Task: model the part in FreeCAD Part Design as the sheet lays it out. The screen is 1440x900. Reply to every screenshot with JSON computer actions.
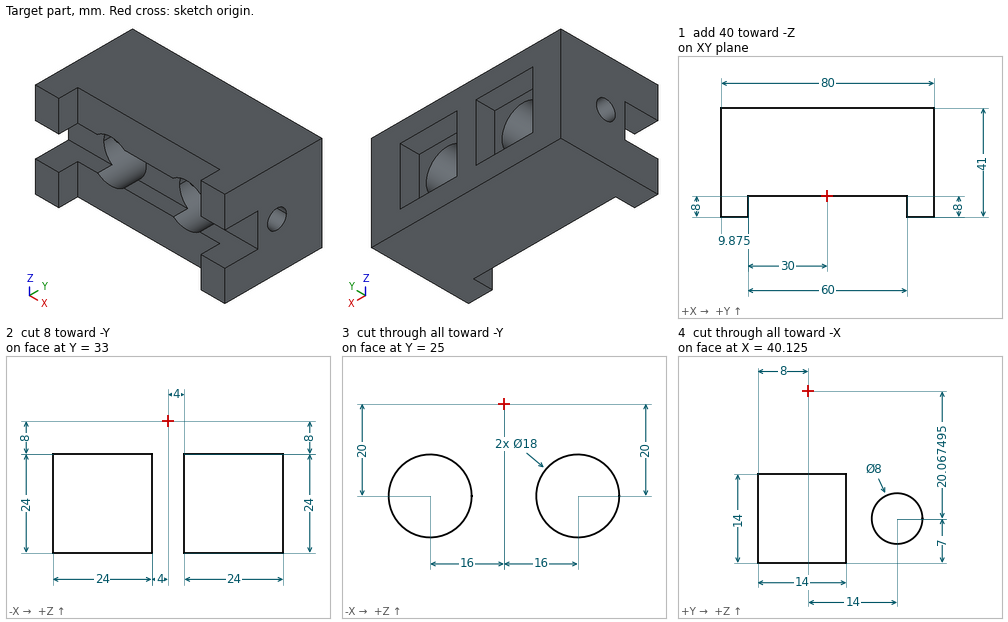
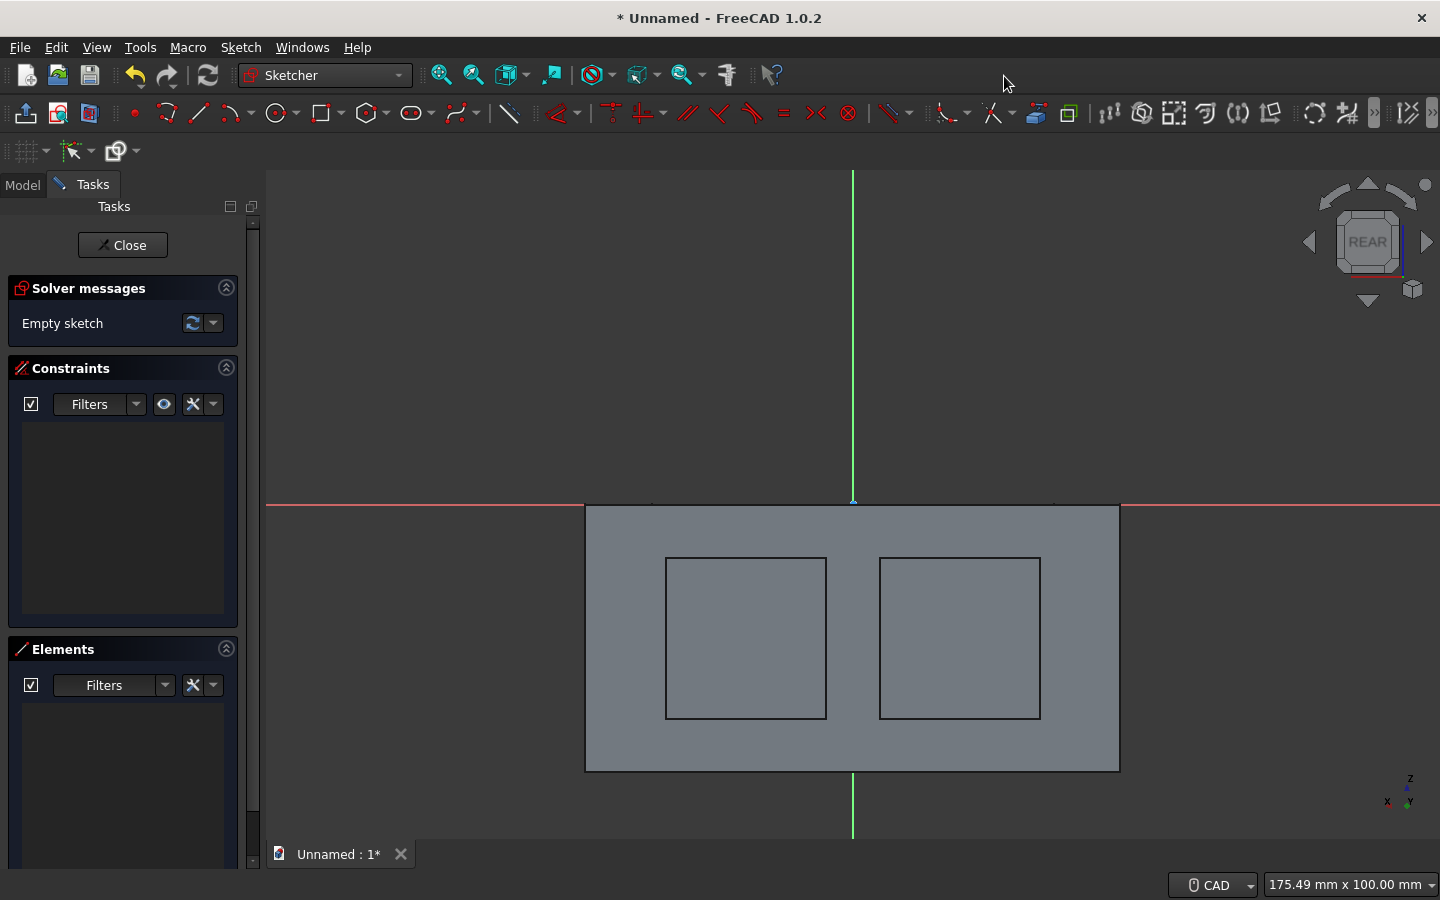
{"action": "scroll", "coordinate": [909, 681], "scroll_direction": "up", "scroll_amount": 4}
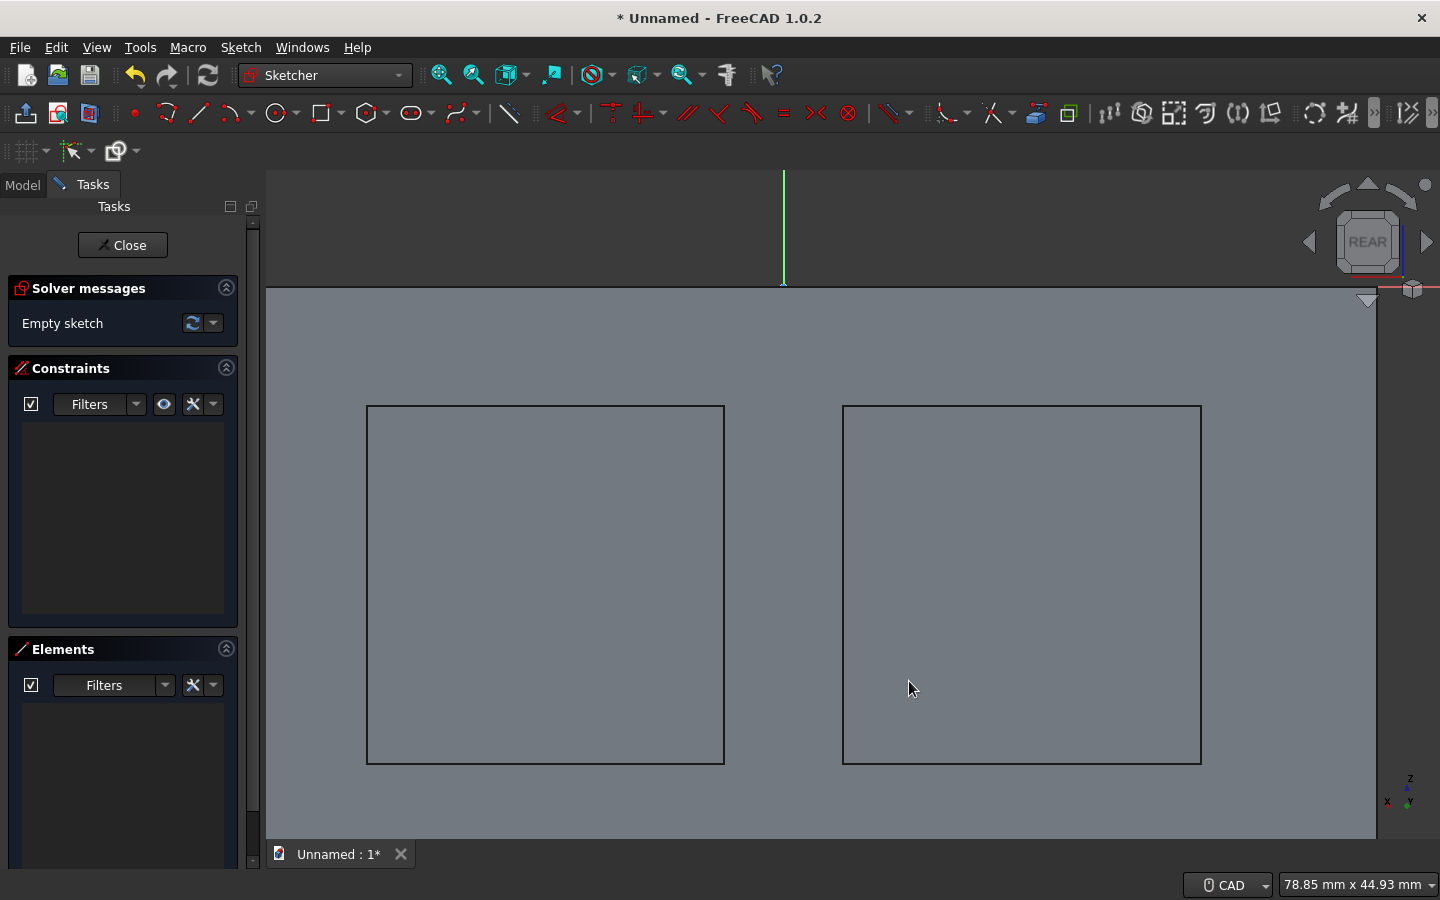
{"action": "left_click", "coordinate": [276, 114]}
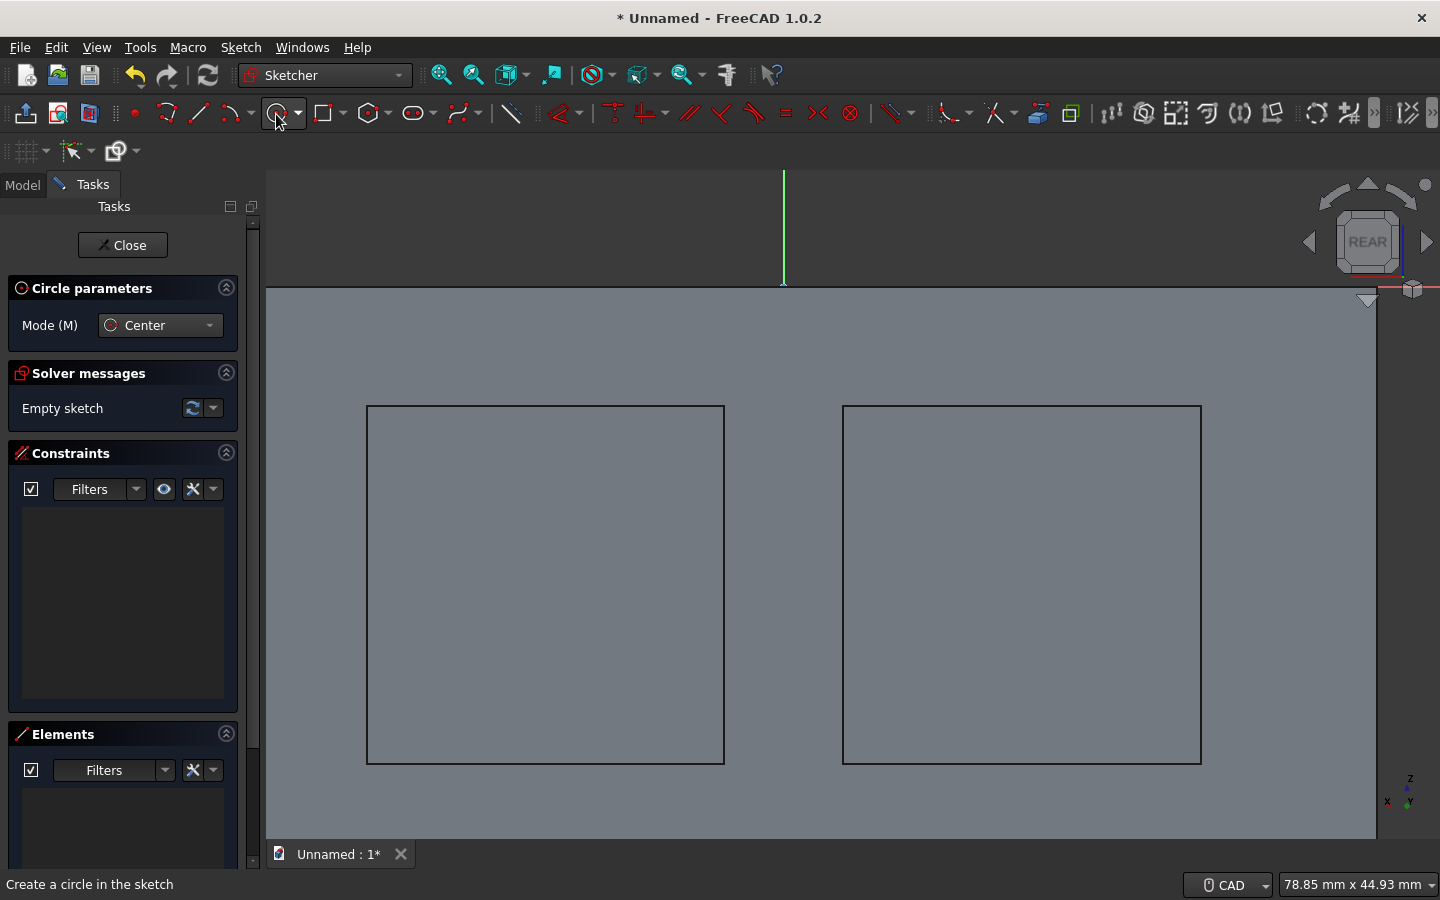
{"action": "left_click", "coordinate": [1022, 585]}
{"action": "left_click", "coordinate": [1117, 490]}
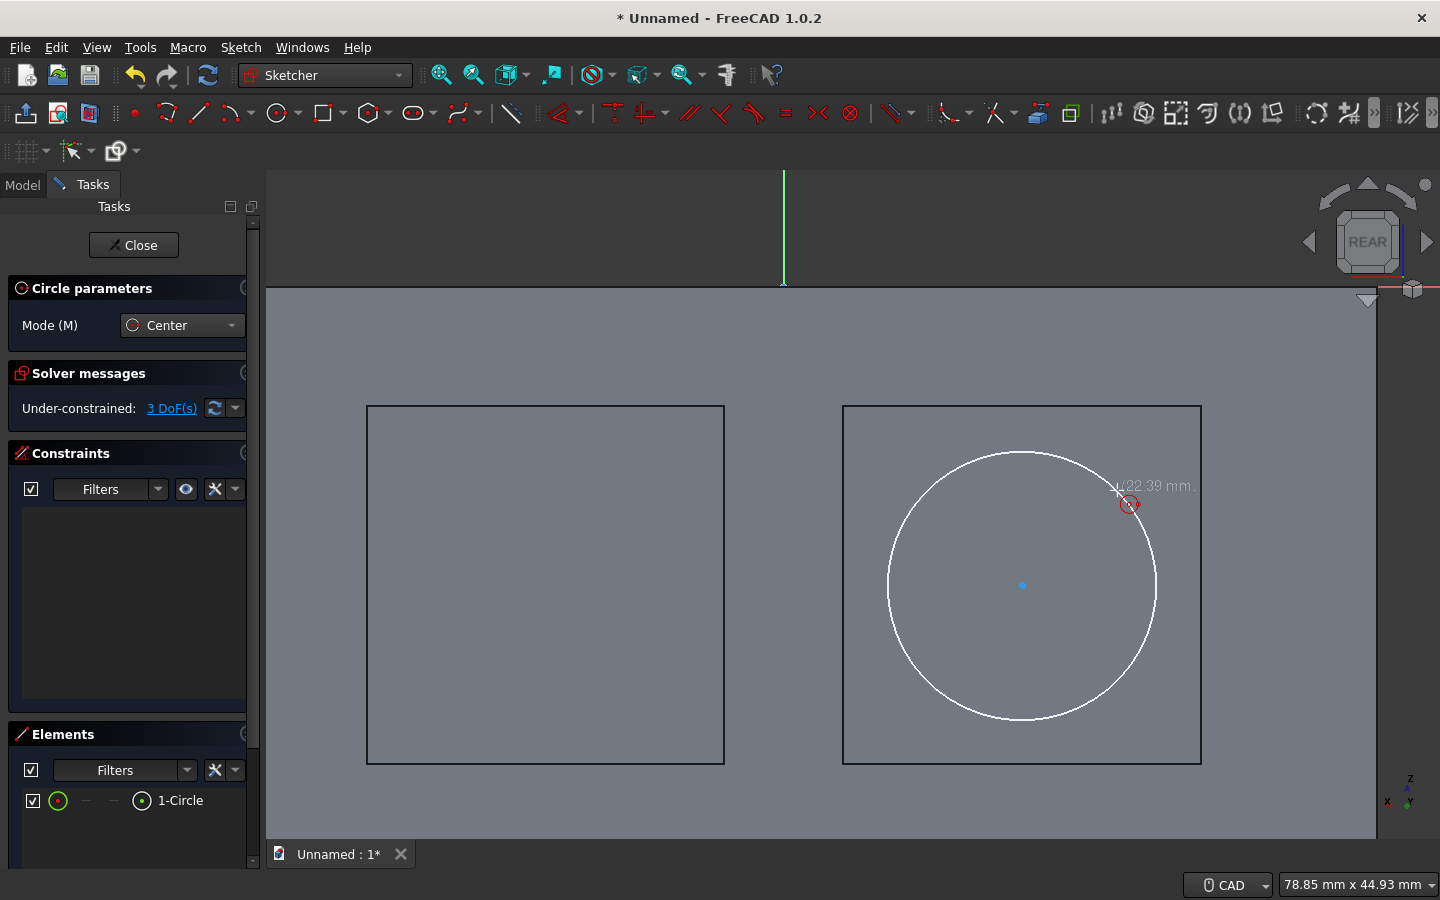
{"action": "left_click", "coordinate": [545, 585]}
{"action": "left_click", "coordinate": [640, 490]}
{"action": "key", "text": "Escape"}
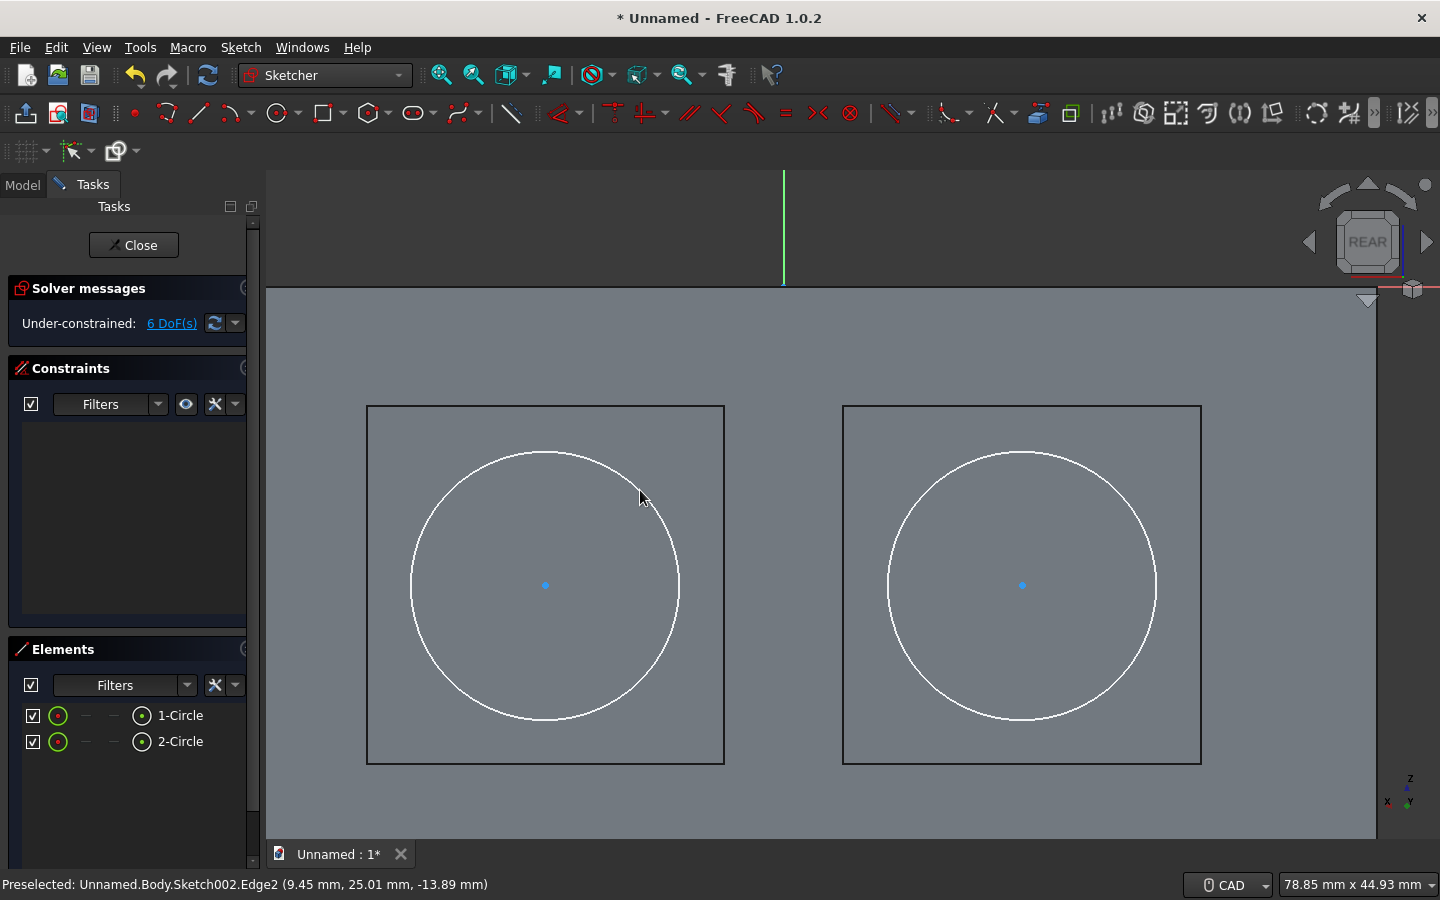
{"action": "left_click", "coordinate": [1117, 491]}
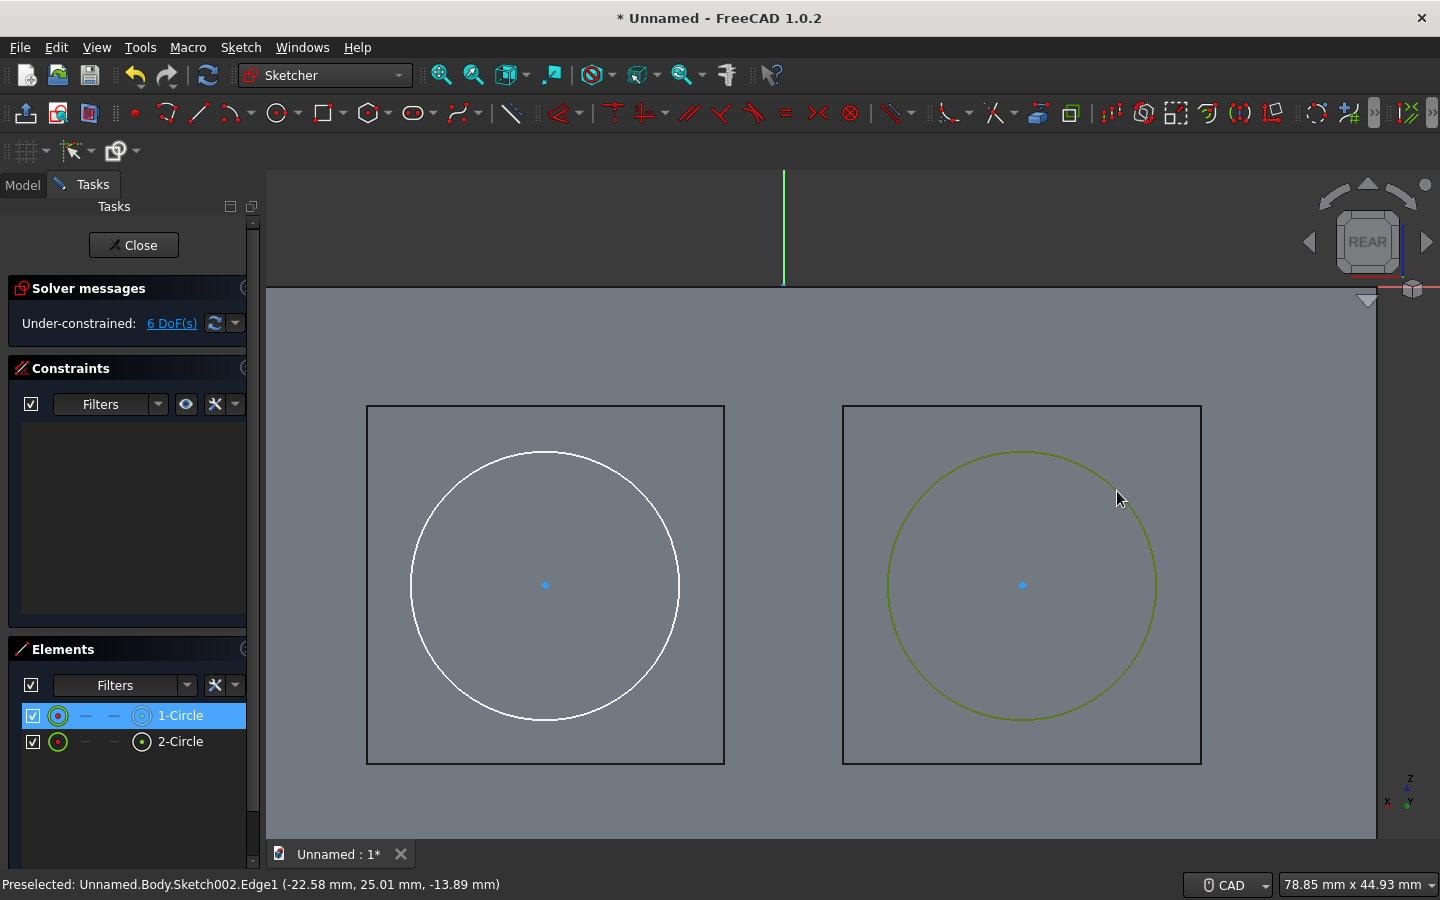
{"action": "left_click", "coordinate": [640, 491]}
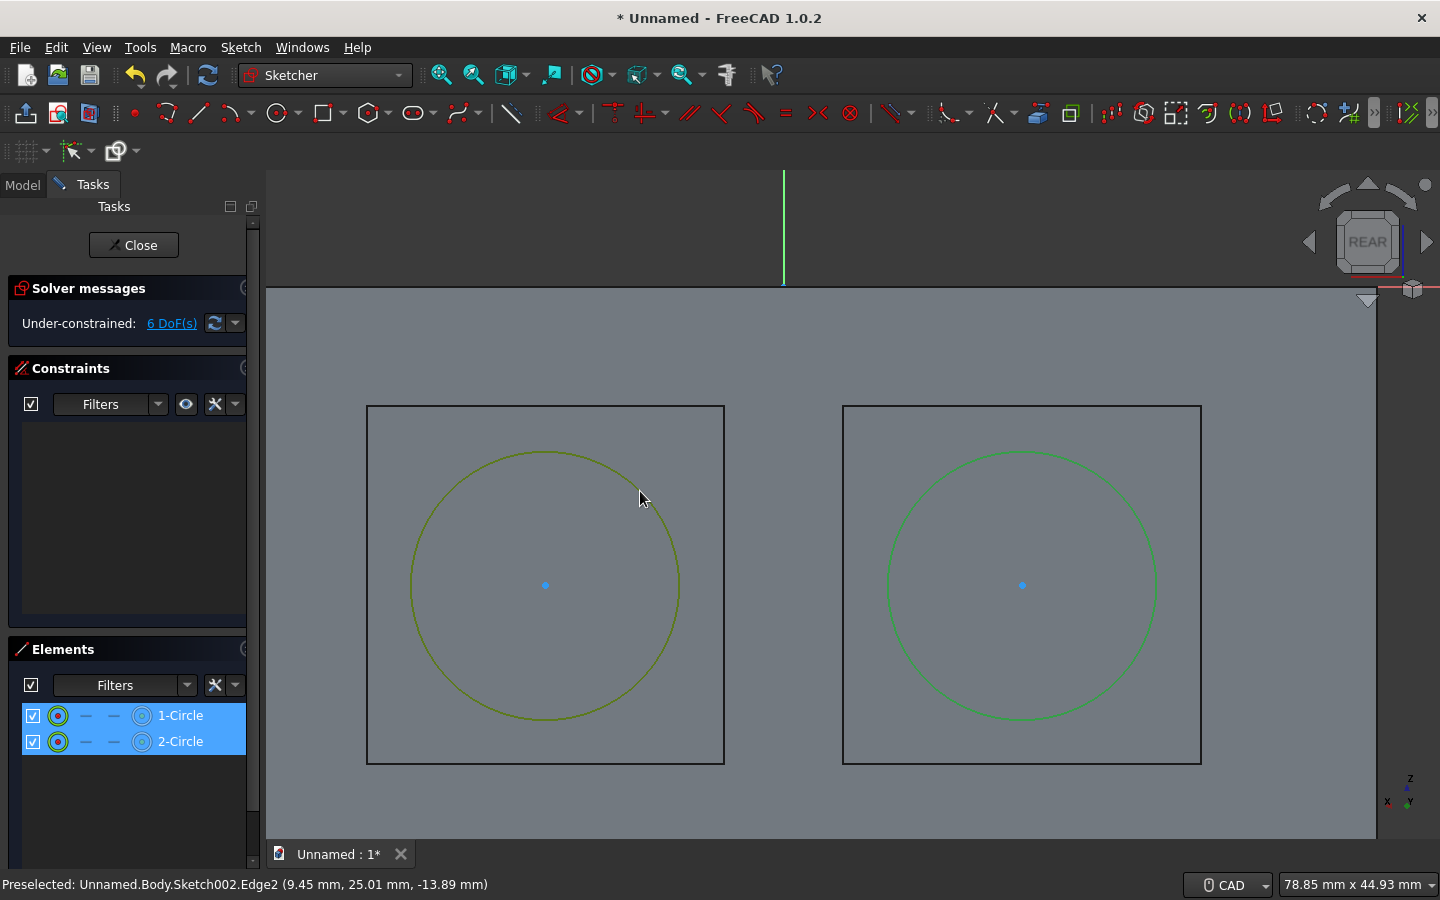
{"action": "left_click", "coordinate": [786, 114]}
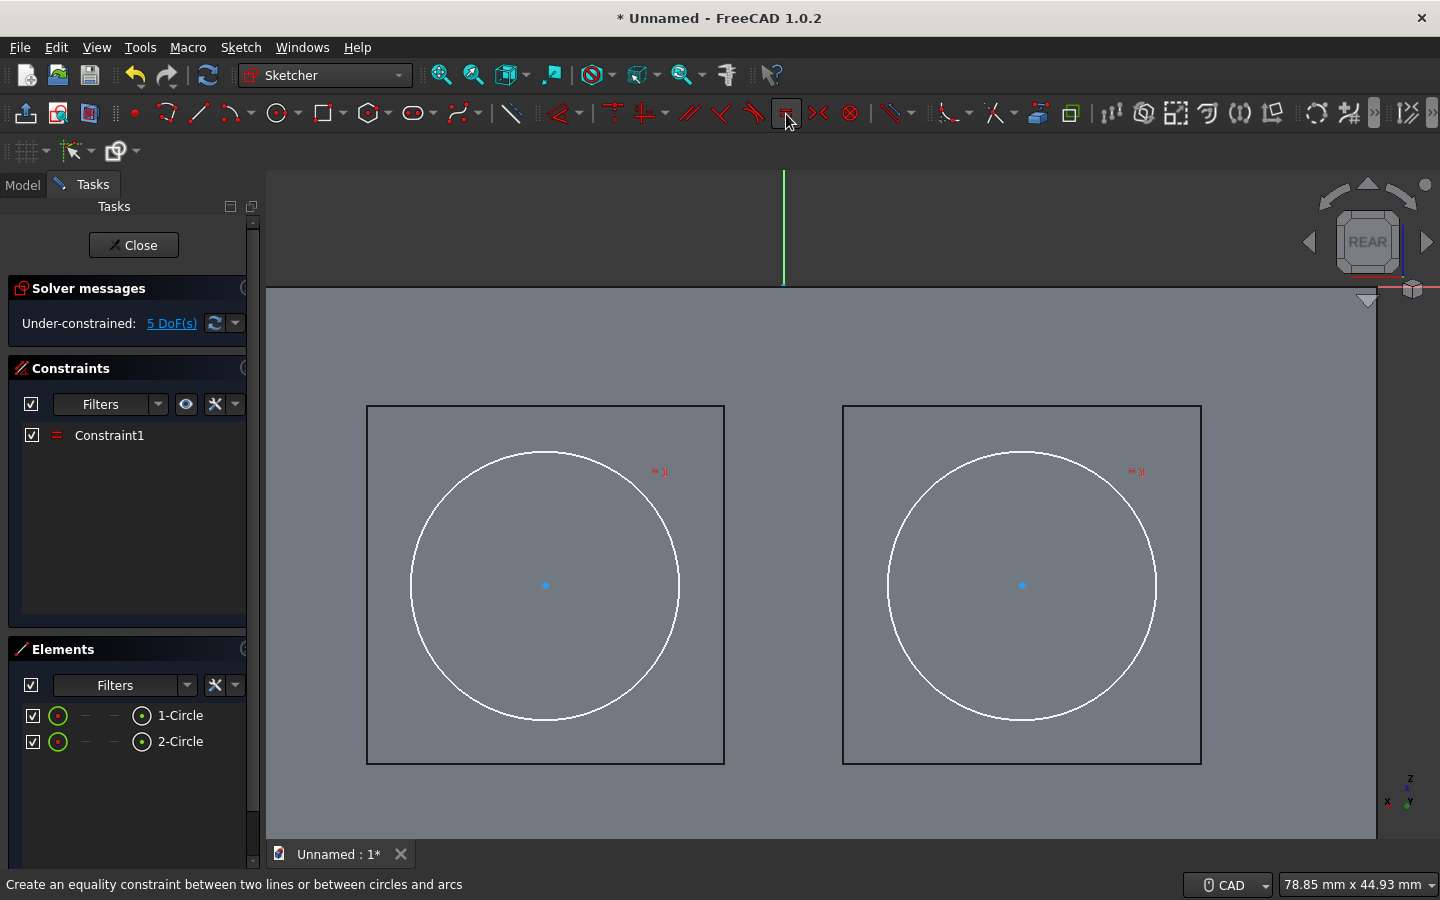
{"action": "left_click", "coordinate": [558, 114]}